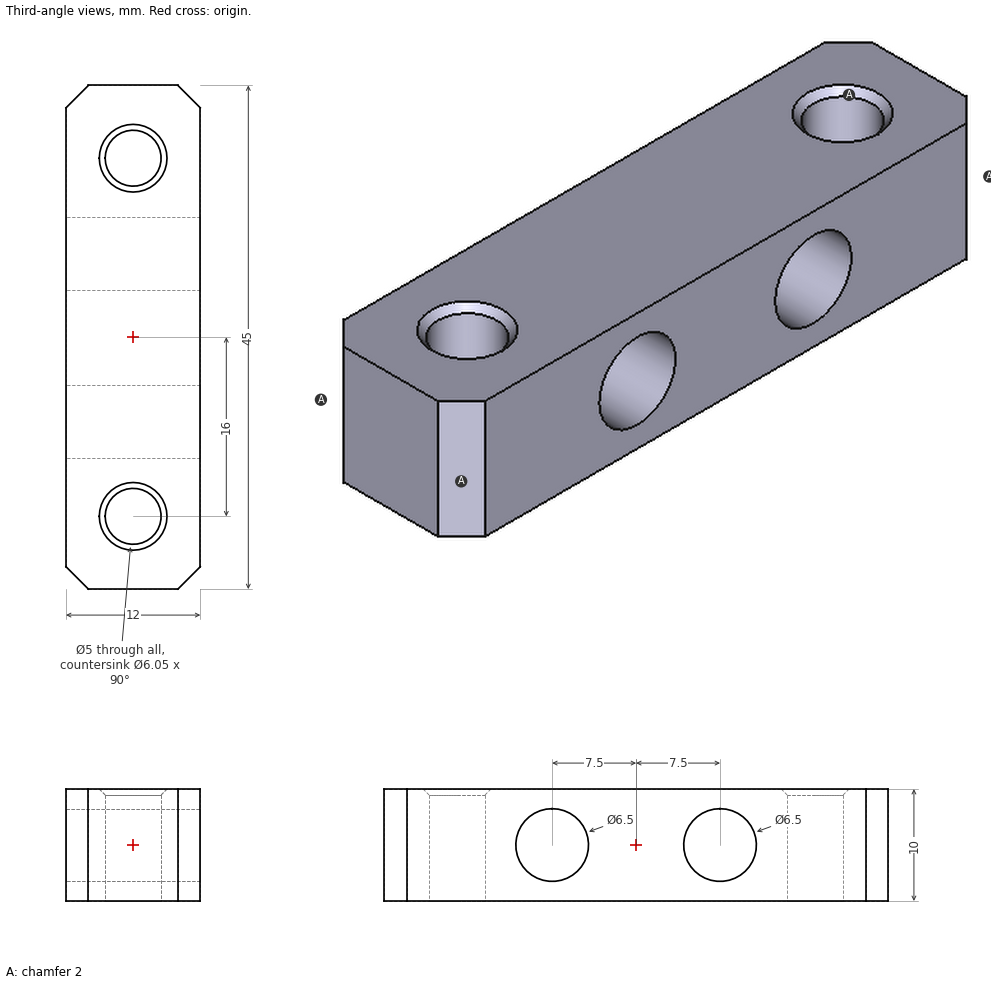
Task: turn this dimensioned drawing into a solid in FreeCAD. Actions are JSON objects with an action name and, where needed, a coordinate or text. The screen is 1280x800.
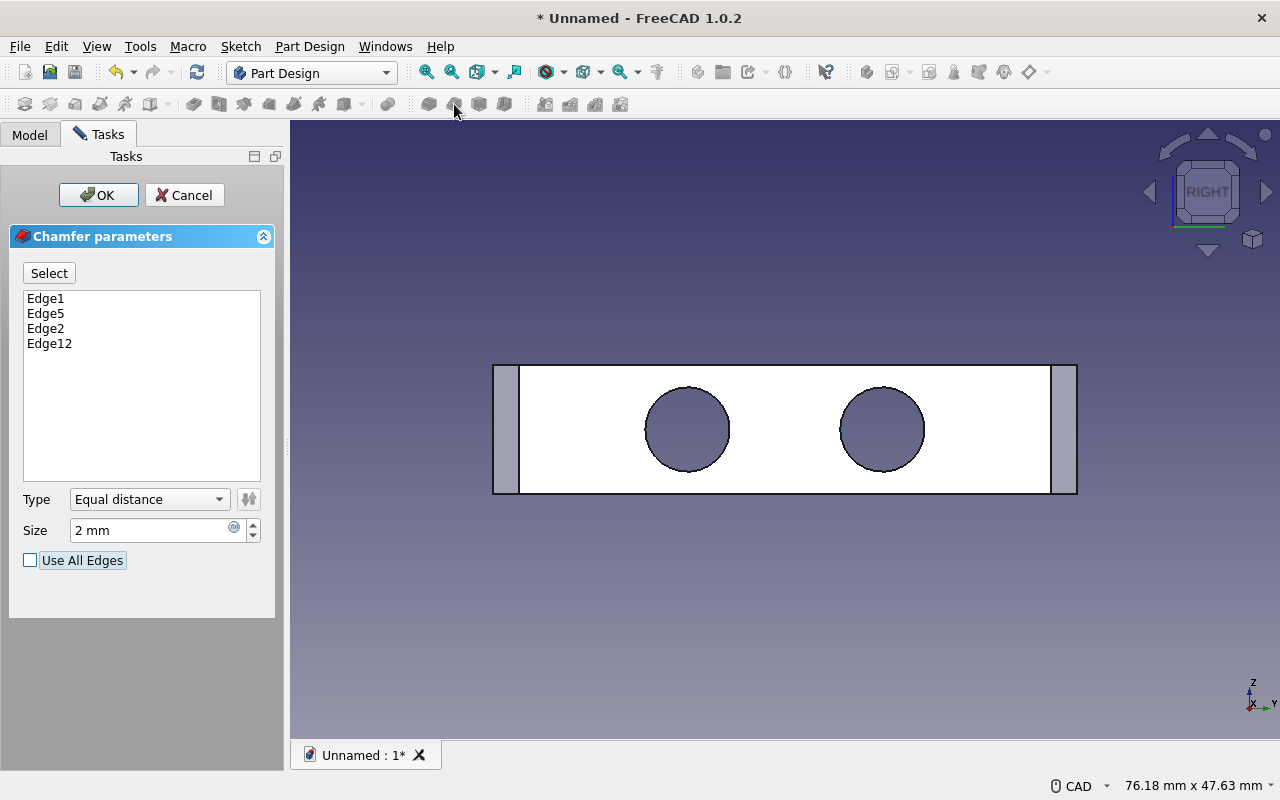
{"action": "left_click", "coordinate": [99, 195]}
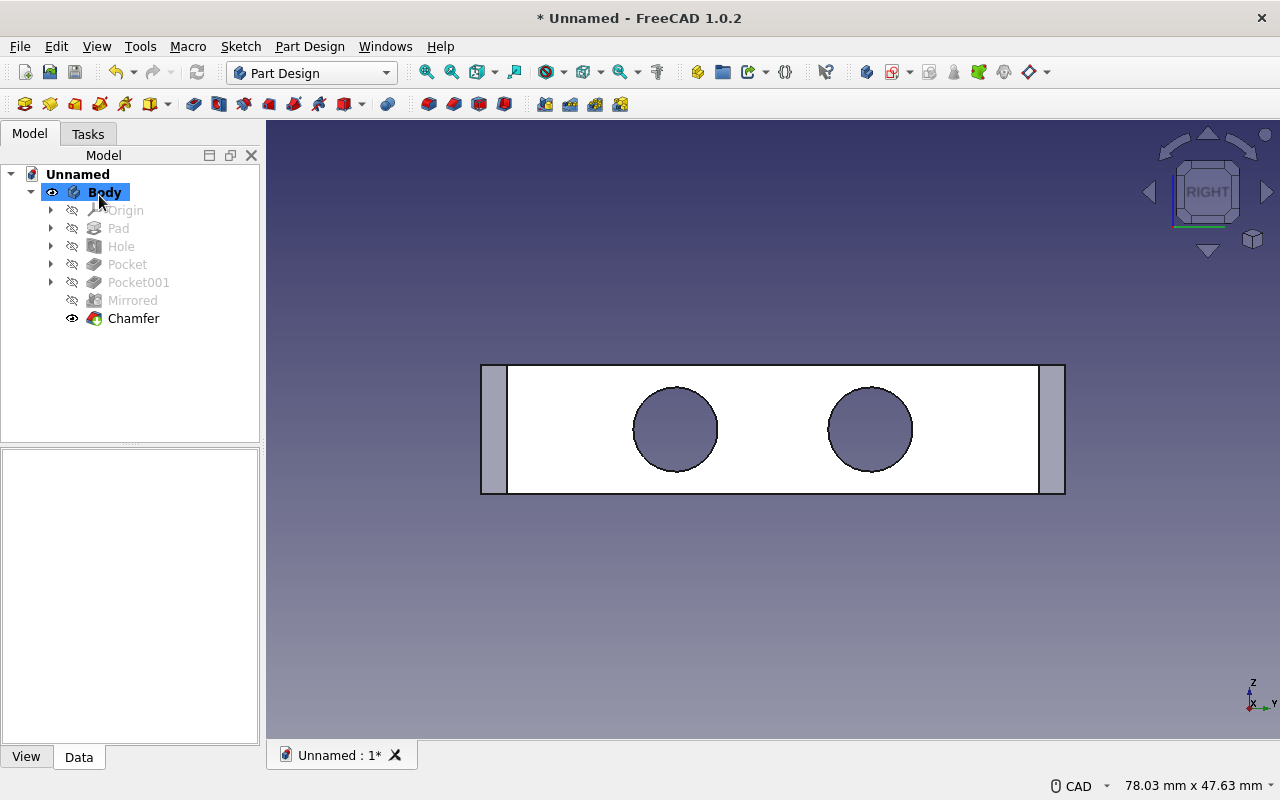
{"action": "key", "text": "0"}